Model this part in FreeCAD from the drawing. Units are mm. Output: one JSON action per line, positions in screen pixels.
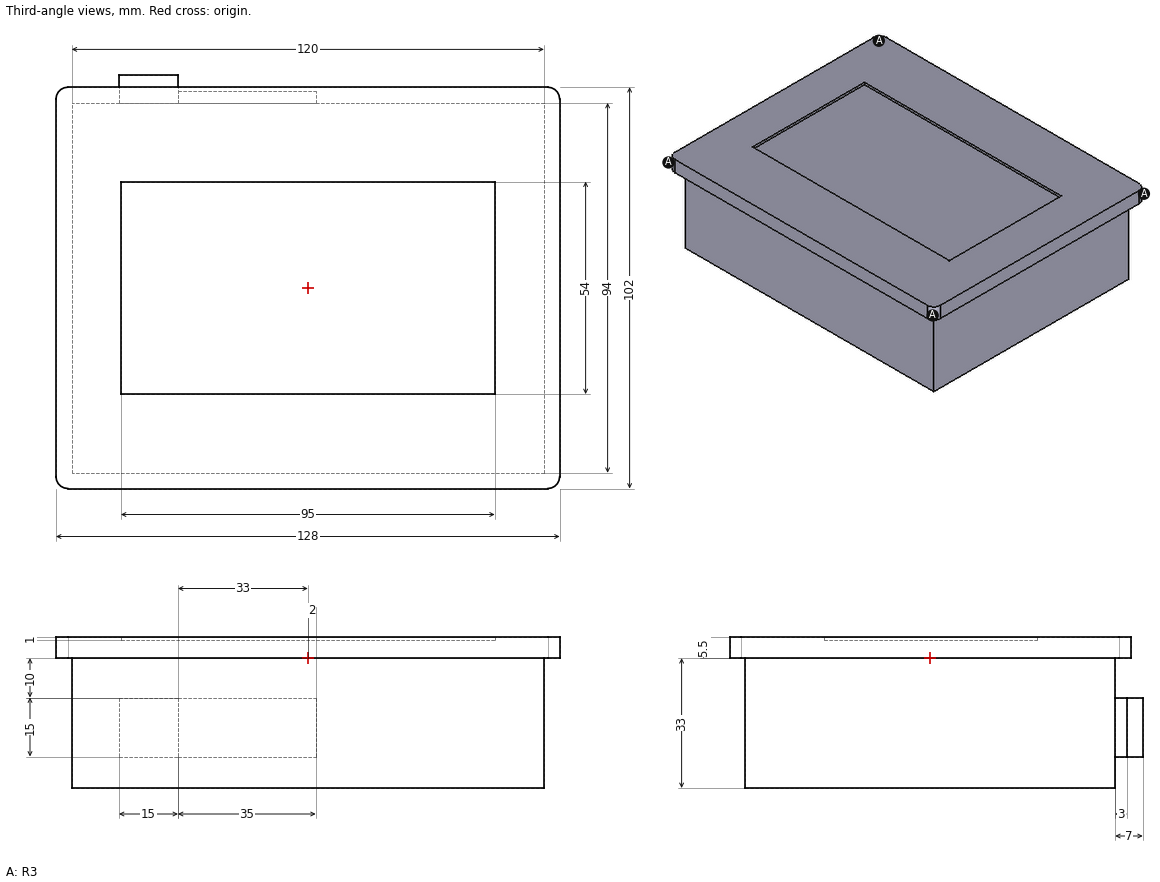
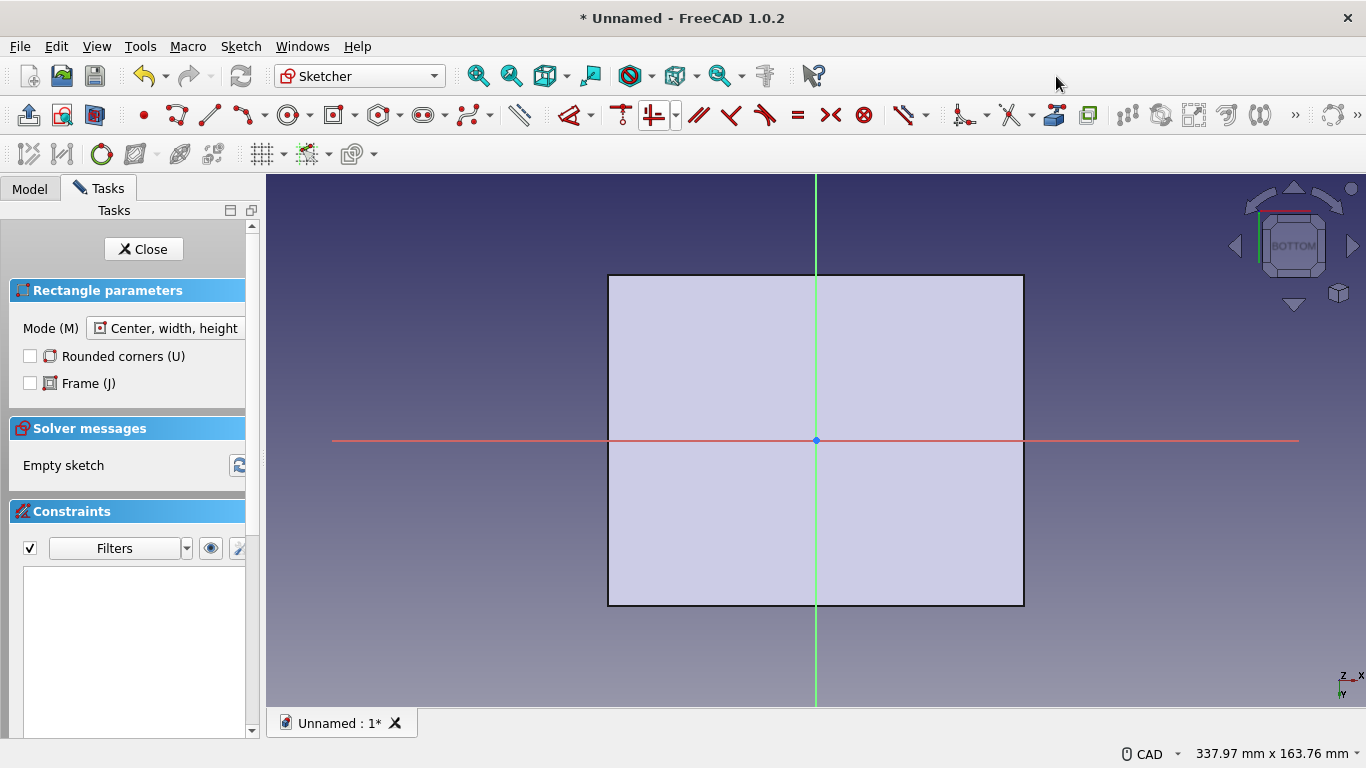
{"action": "left_click", "coordinate": [816, 440]}
{"action": "mouse_move", "coordinate": [1011, 288]}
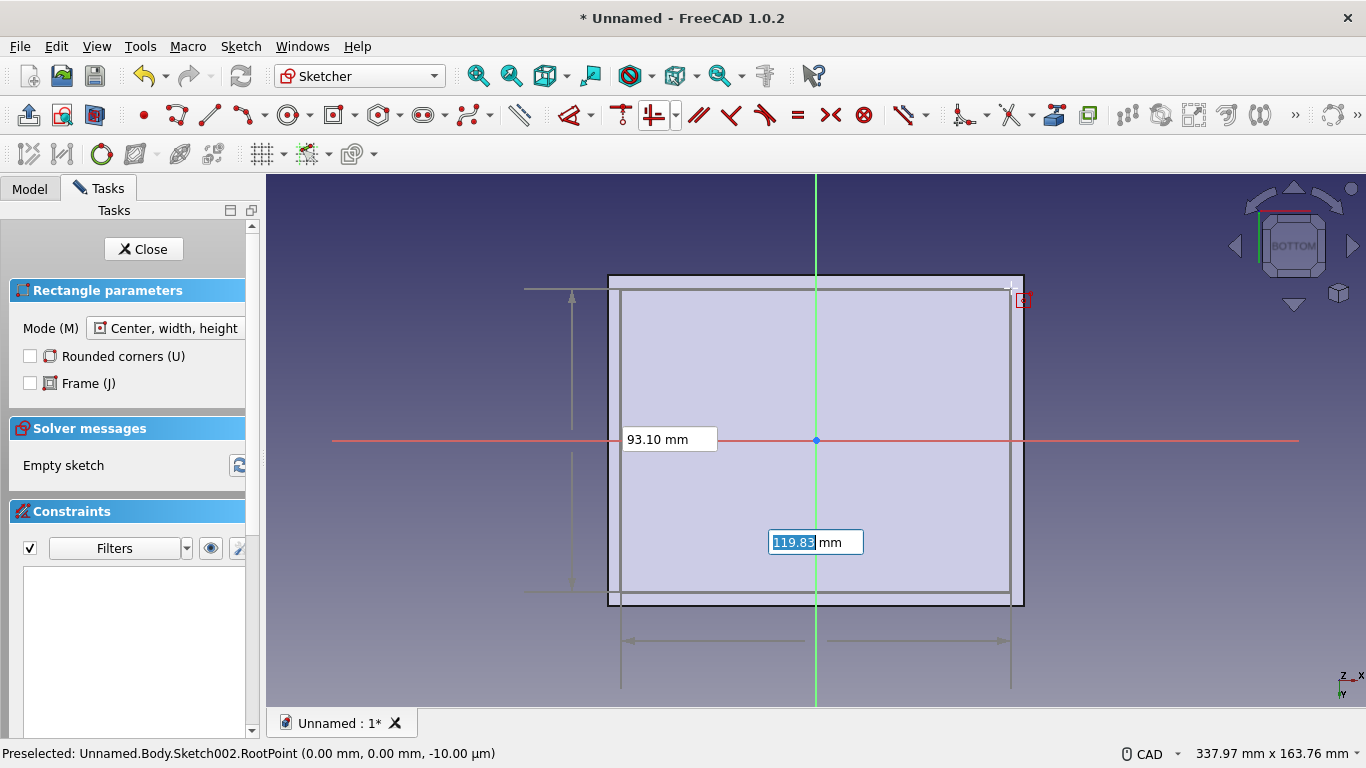
{"action": "type", "text": "120"}
{"action": "key", "text": "Tab"}
{"action": "type", "text": "94"}
{"action": "key", "text": "Return"}
{"action": "key", "text": "Escape"}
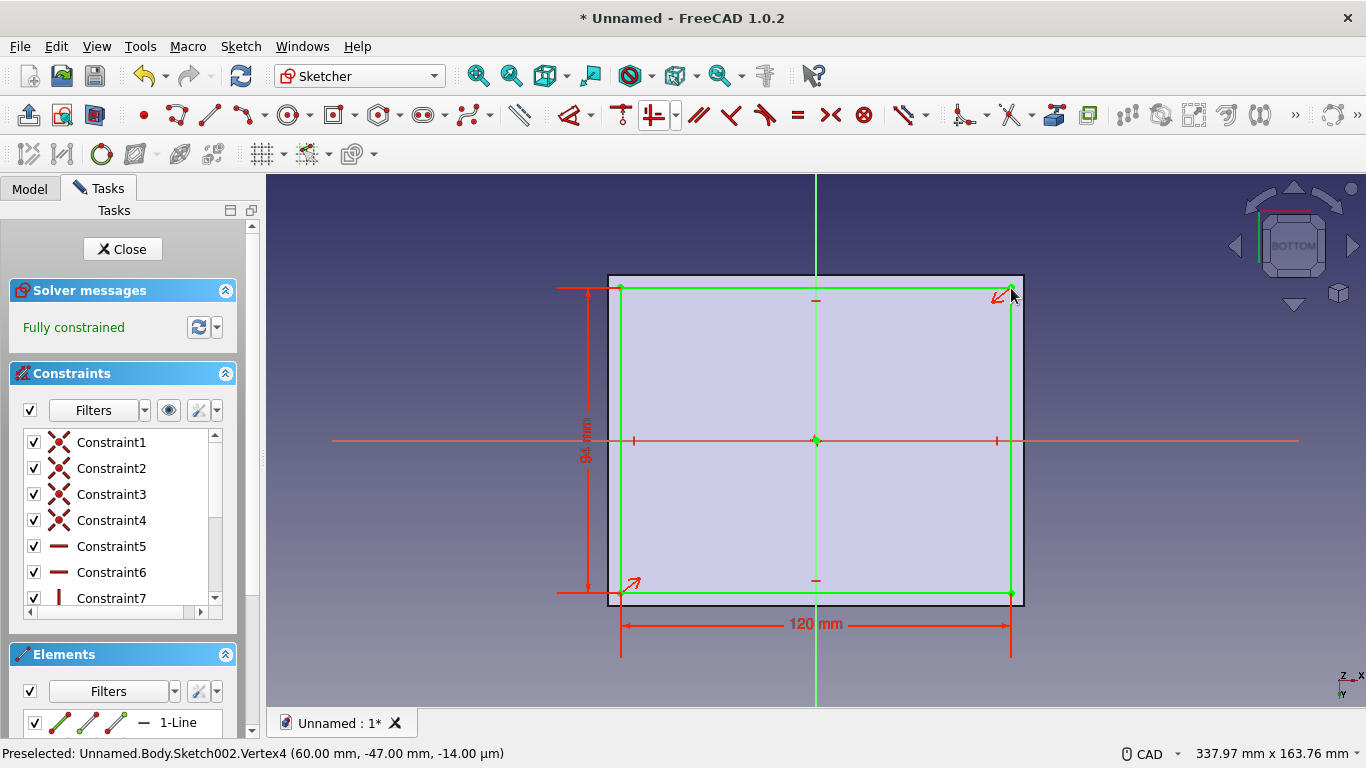
{"action": "left_click", "coordinate": [123, 249]}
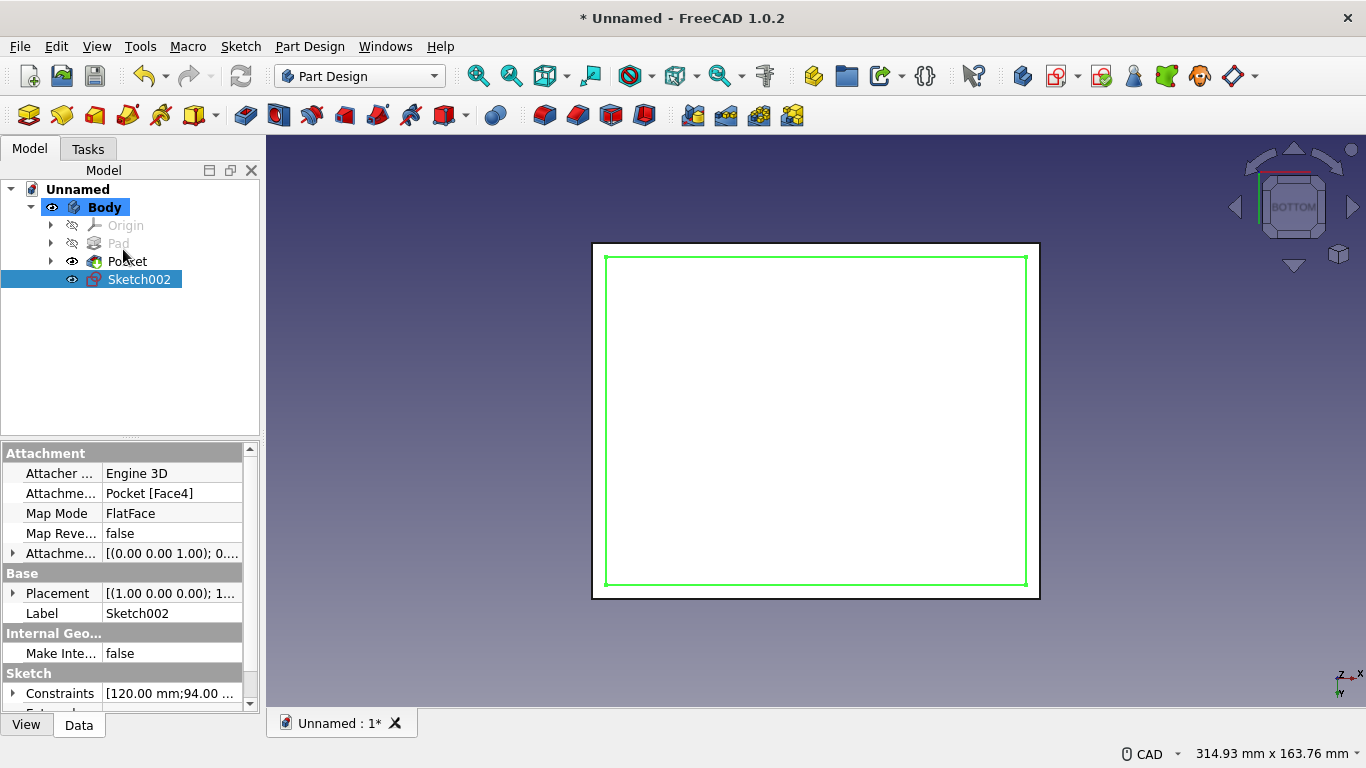
{"action": "left_click", "coordinate": [29, 116]}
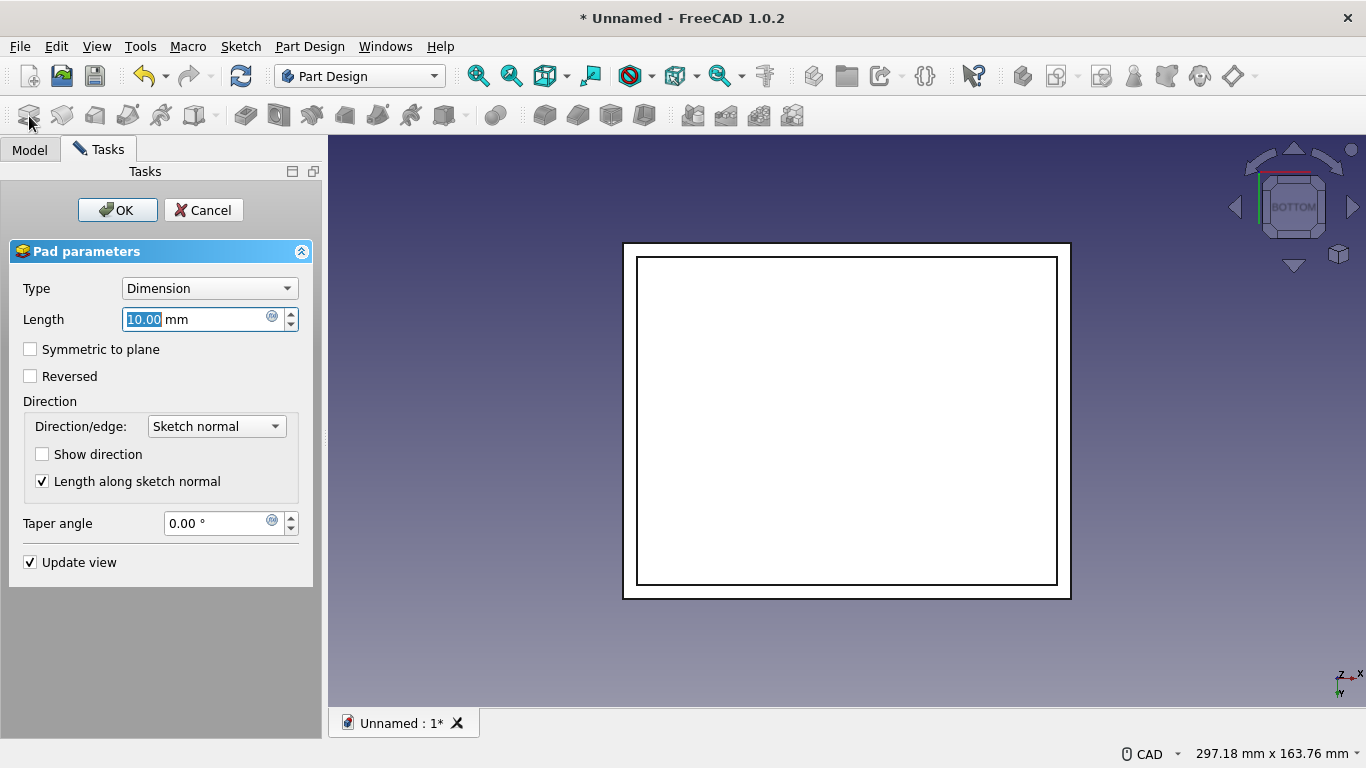
{"action": "type", "text": "33"}
{"action": "key", "text": "Tab"}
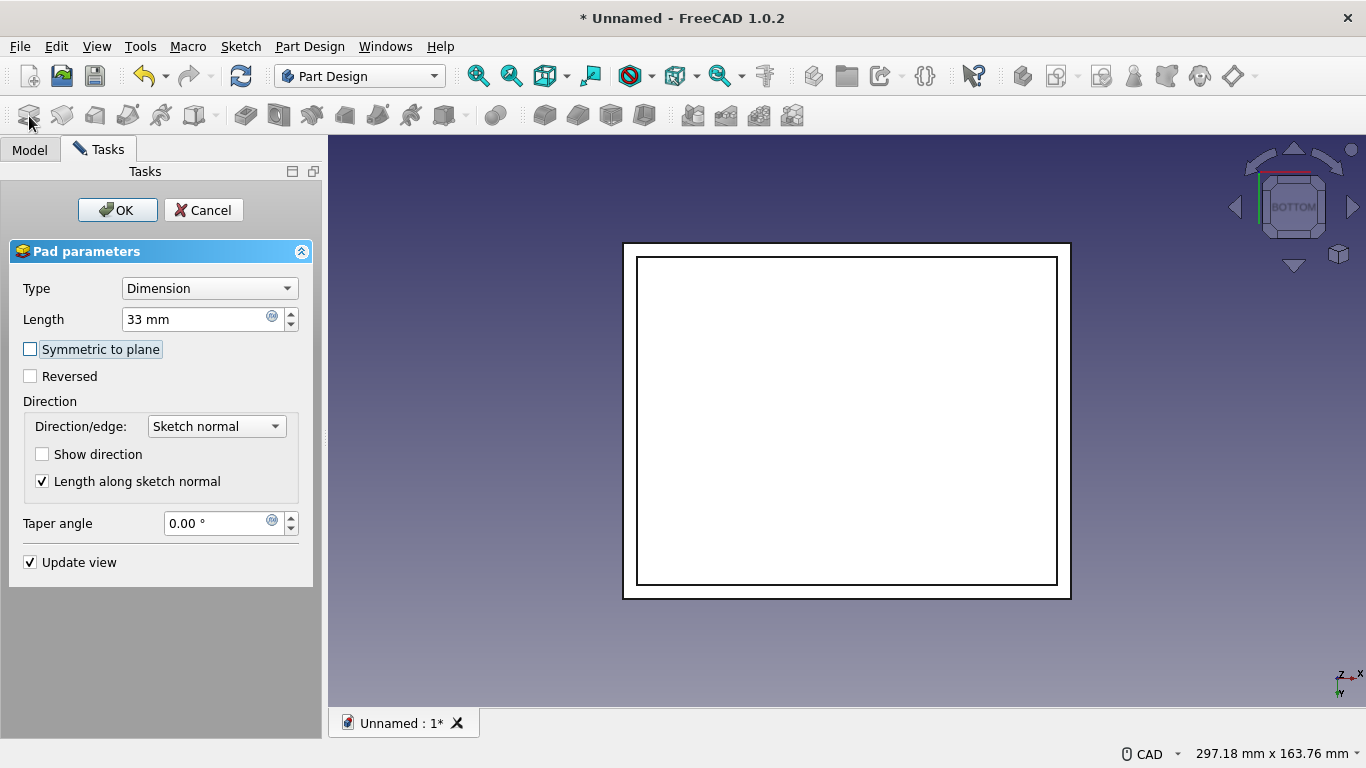
{"action": "left_click", "coordinate": [118, 210]}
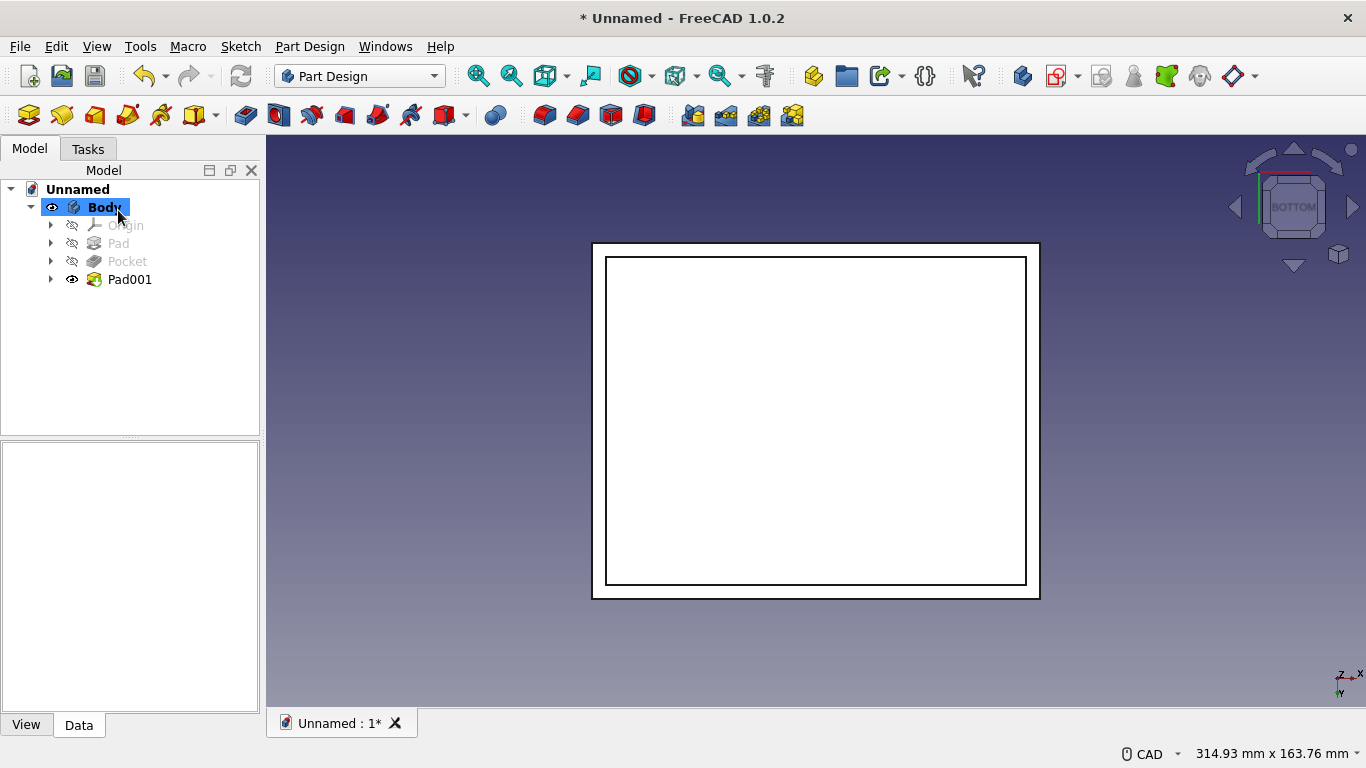
{"action": "scroll", "coordinate": [592, 598], "scroll_direction": "up", "scroll_amount": 4}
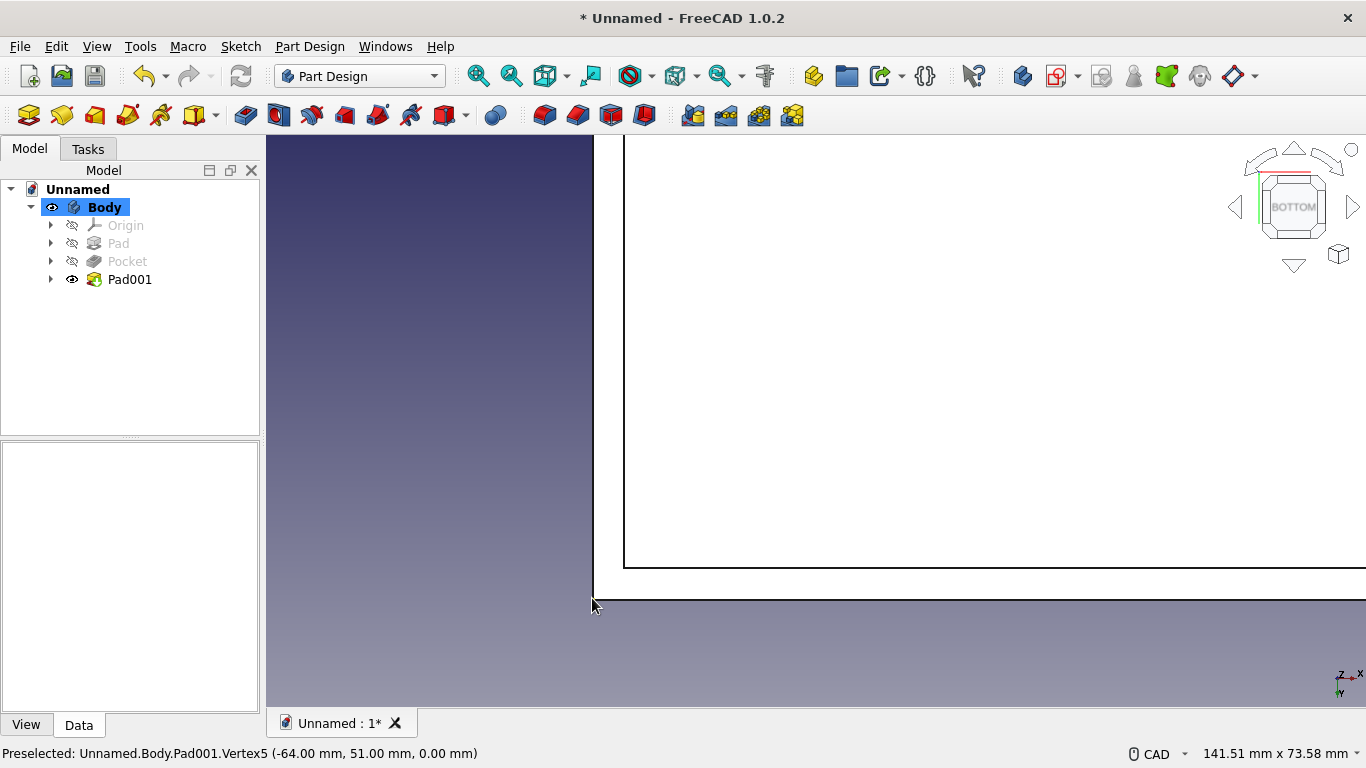
{"action": "key", "text": "v f"}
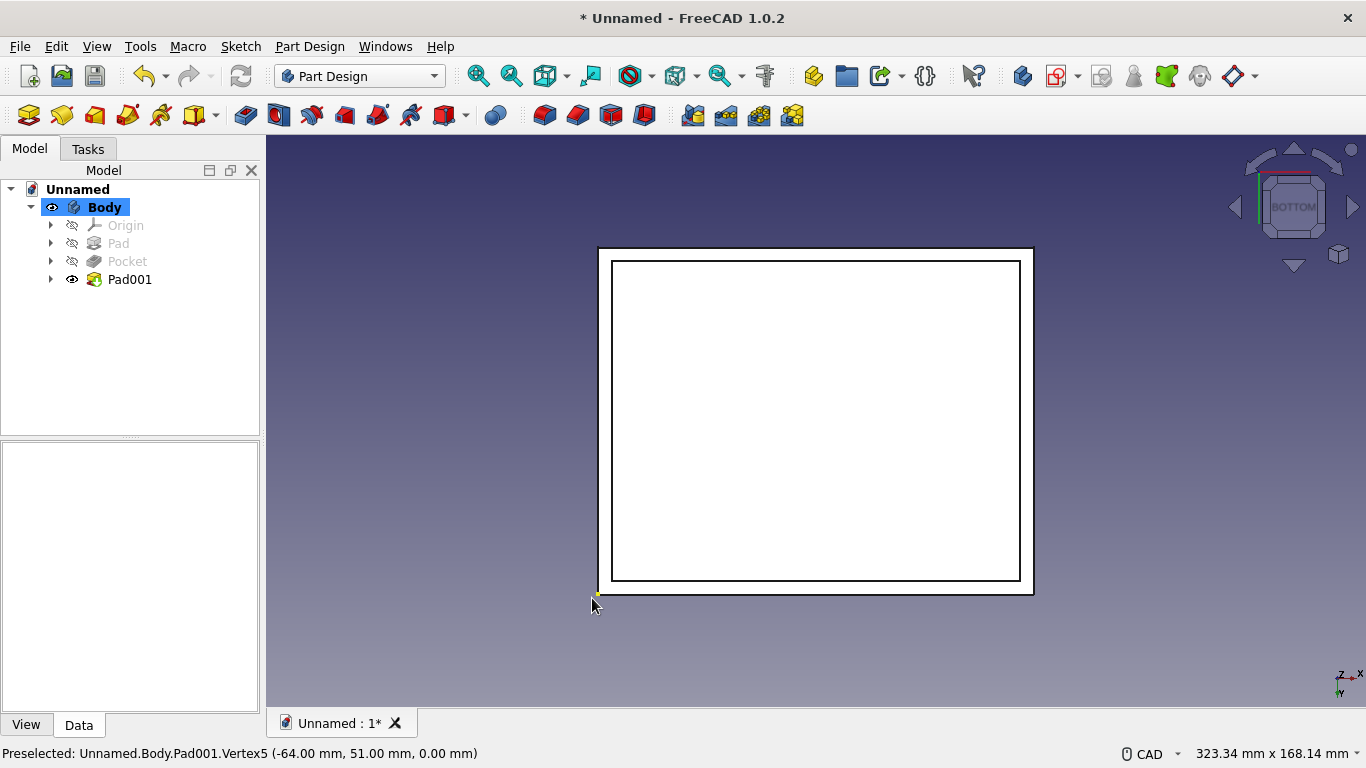
{"action": "key", "text": "0"}